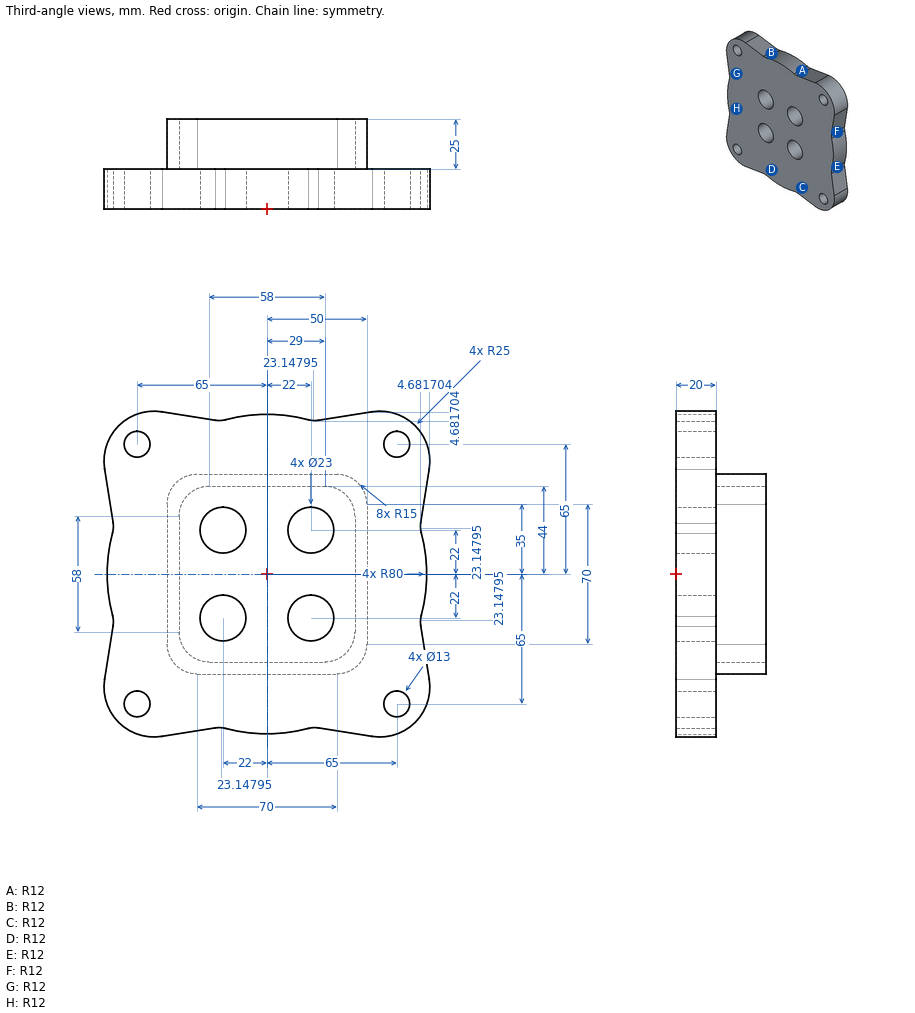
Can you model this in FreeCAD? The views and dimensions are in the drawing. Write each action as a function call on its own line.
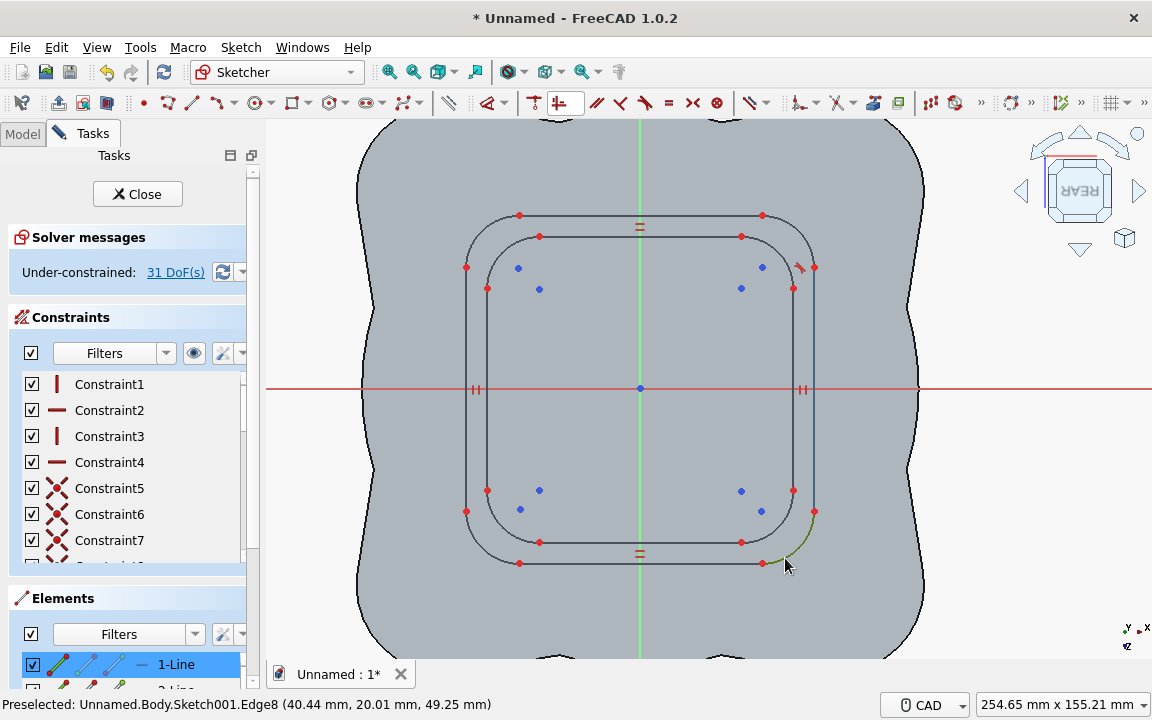
click(646, 104)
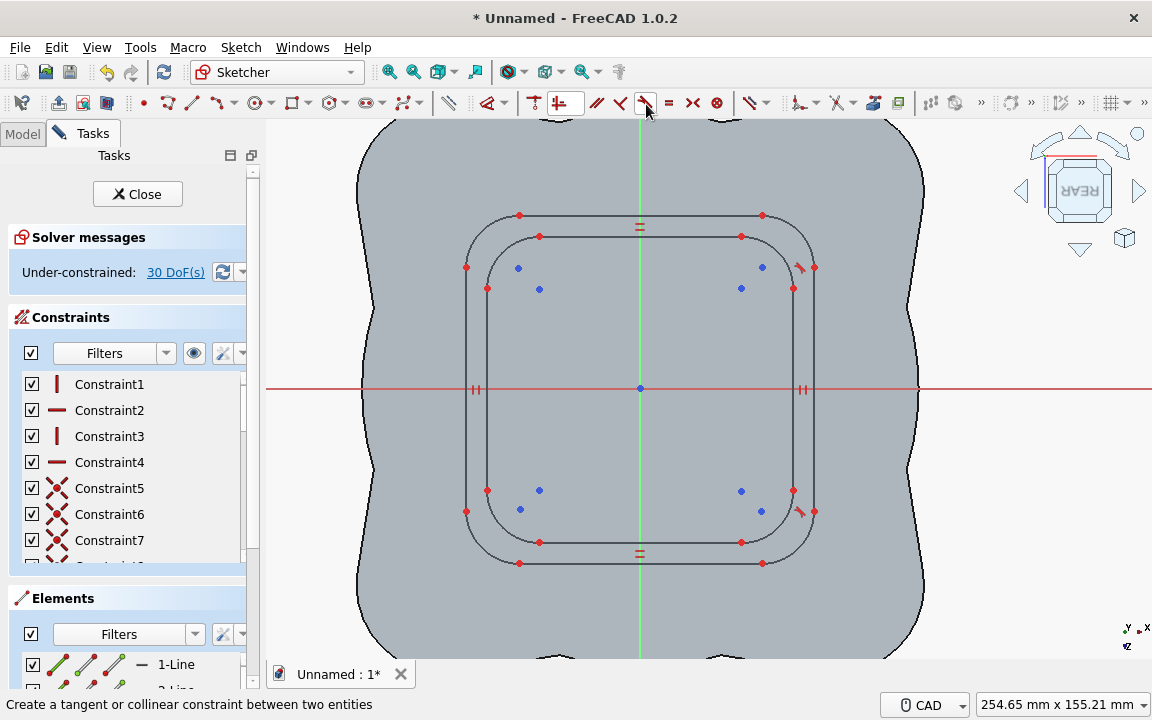
click(689, 216)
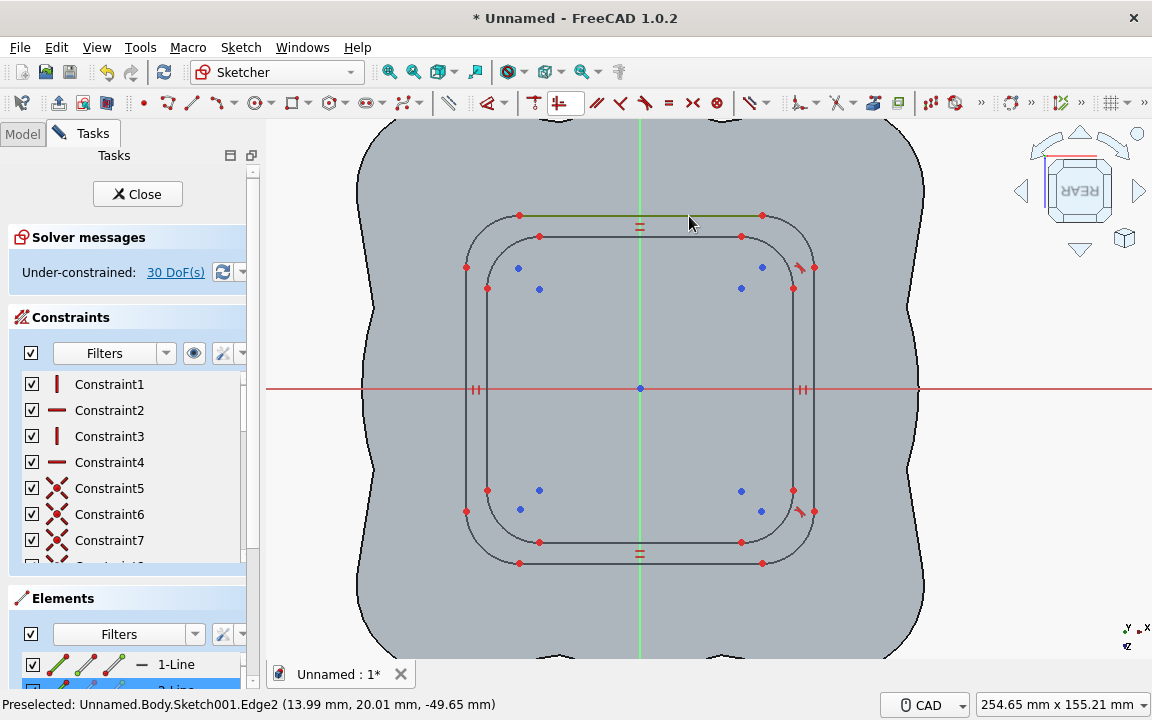
click(808, 244)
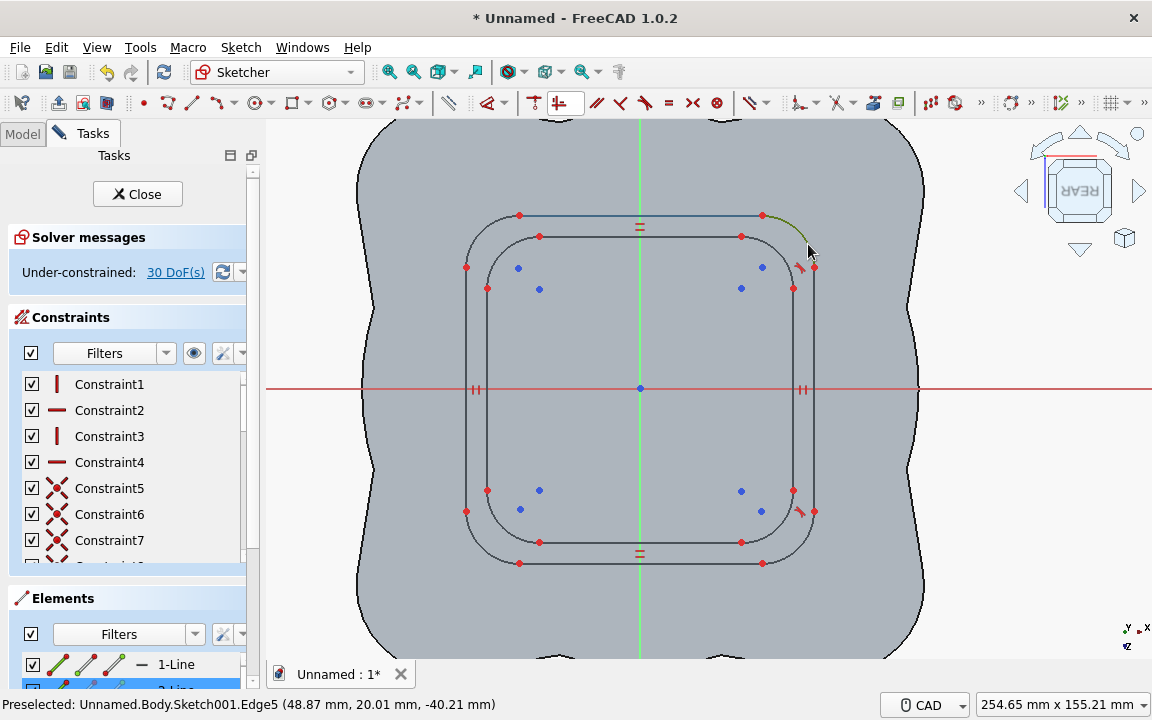
click(646, 104)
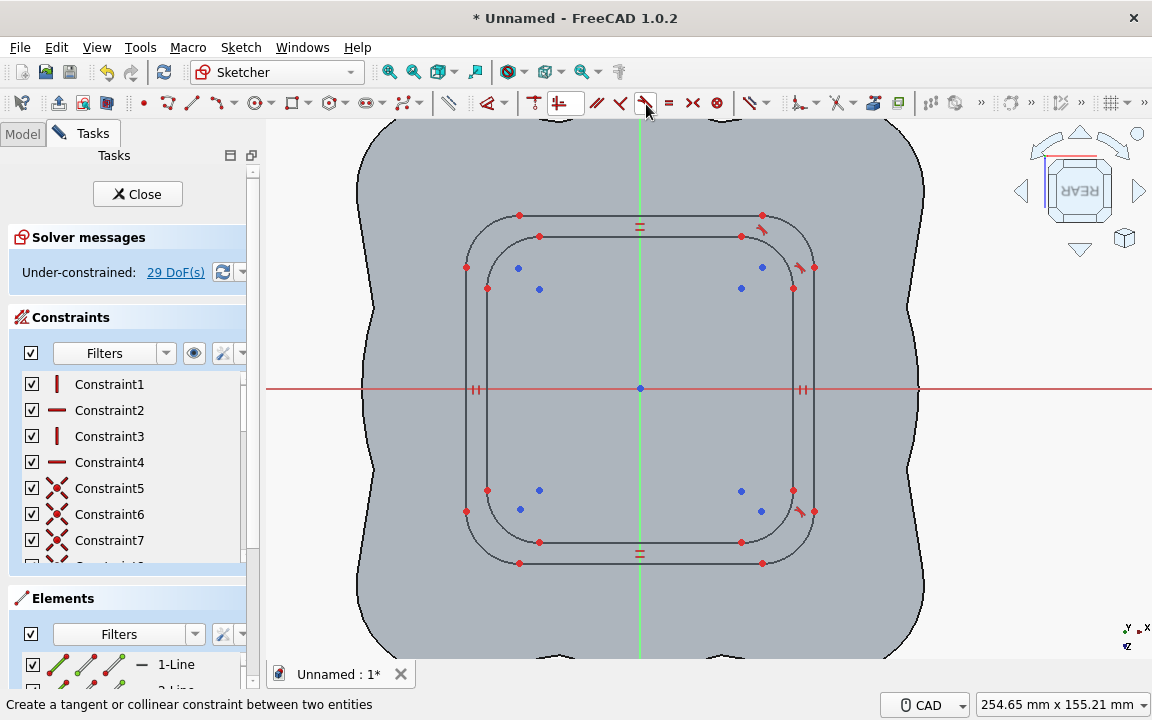
click(689, 216)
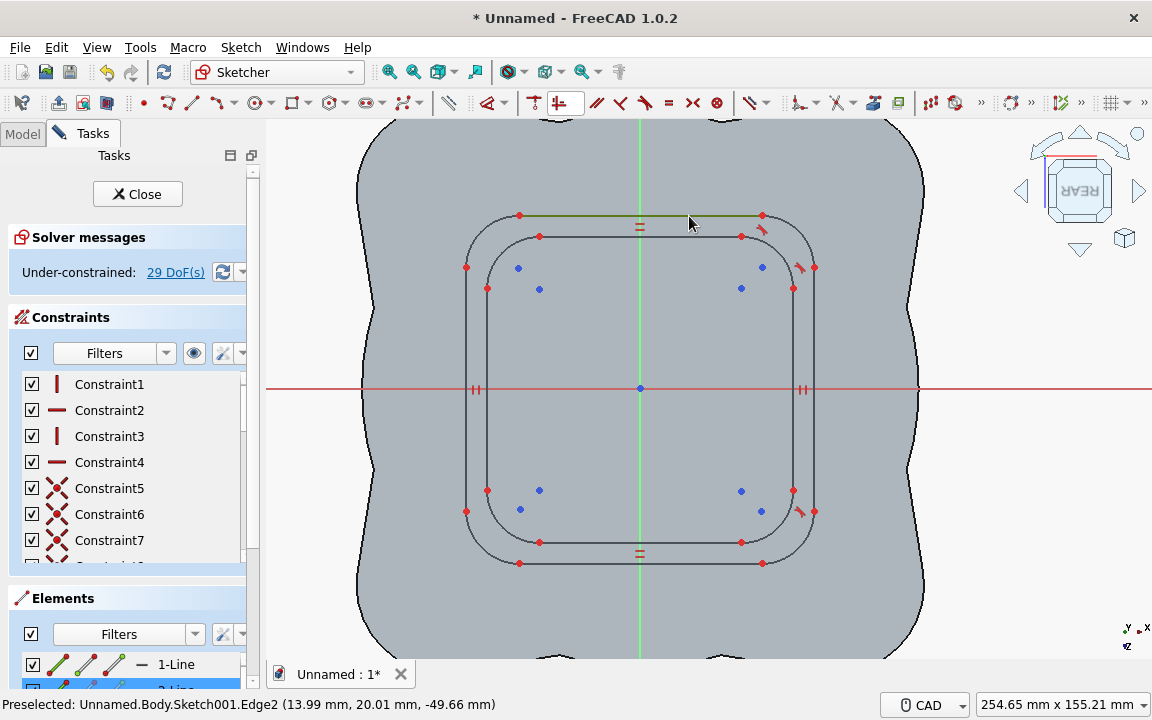
click(495, 222)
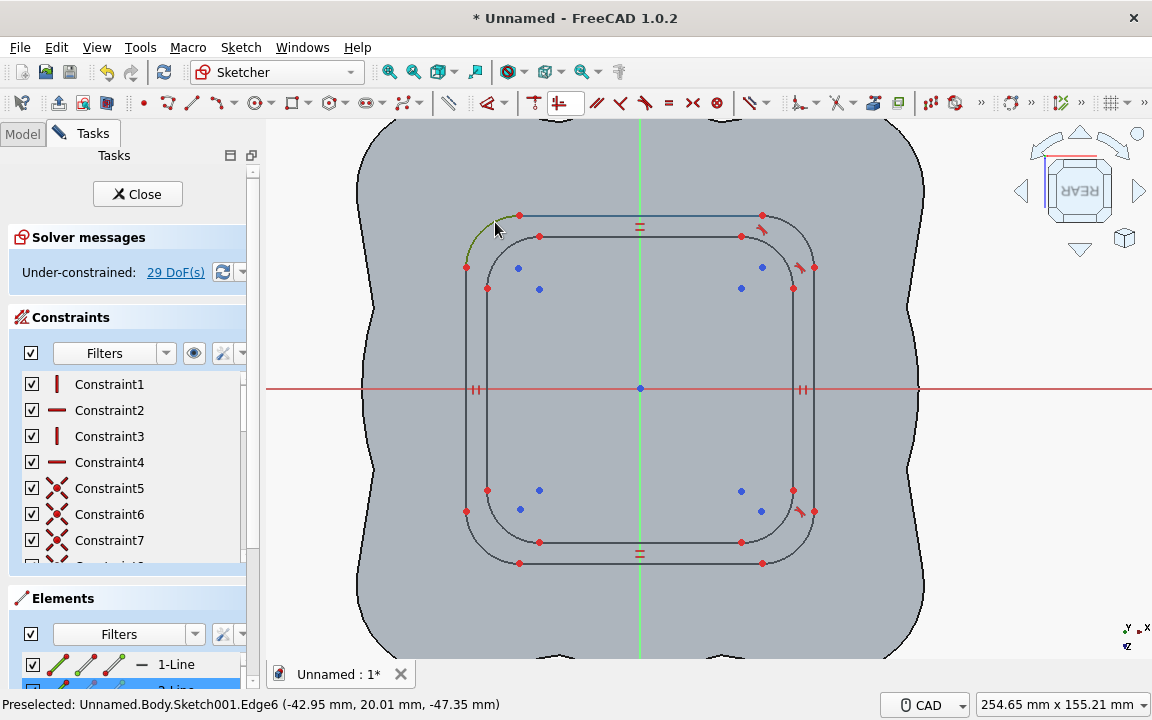
click(646, 104)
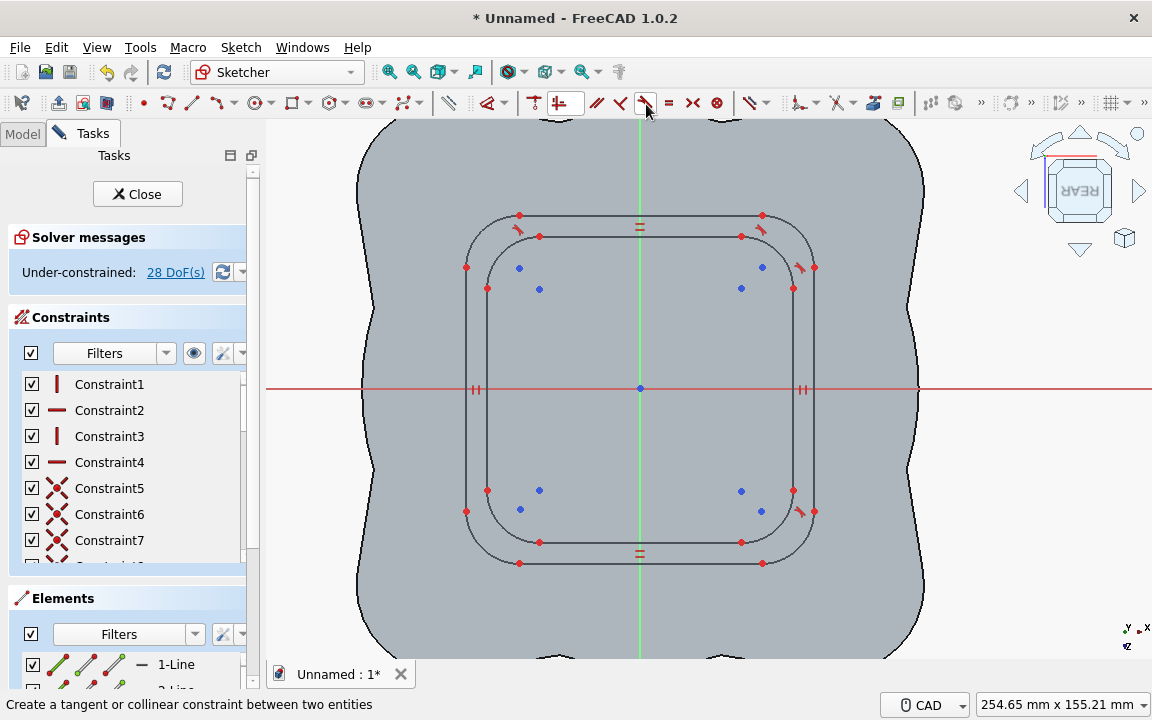
click(466, 341)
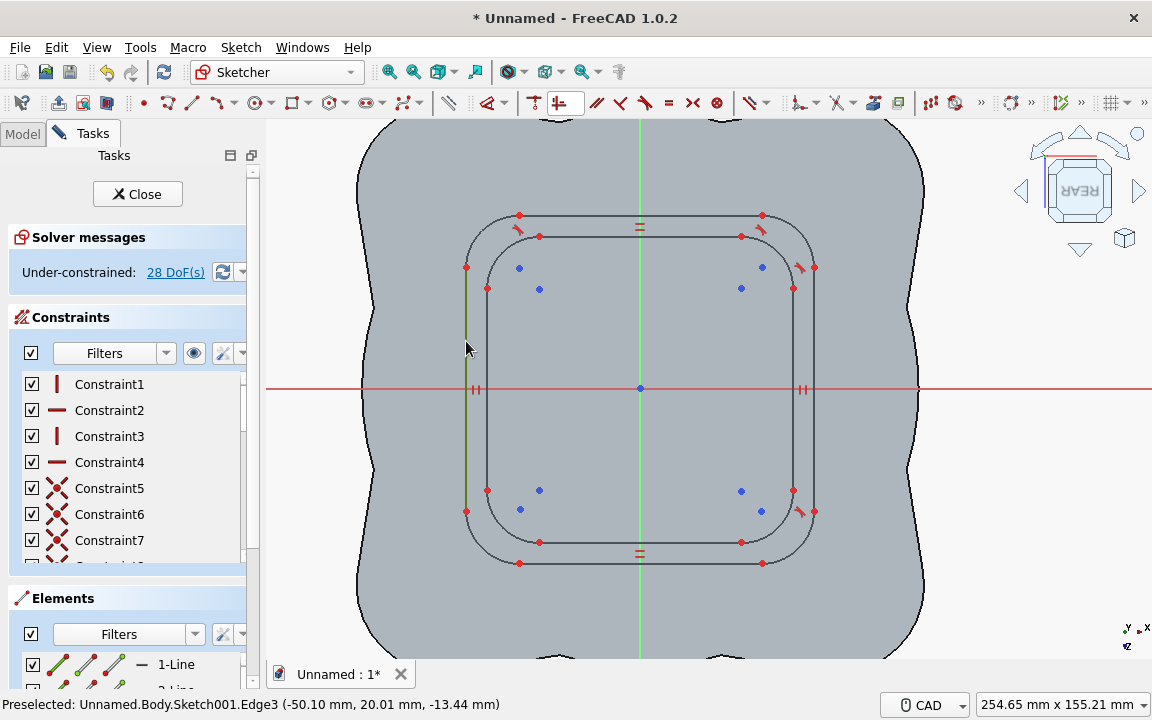
click(495, 222)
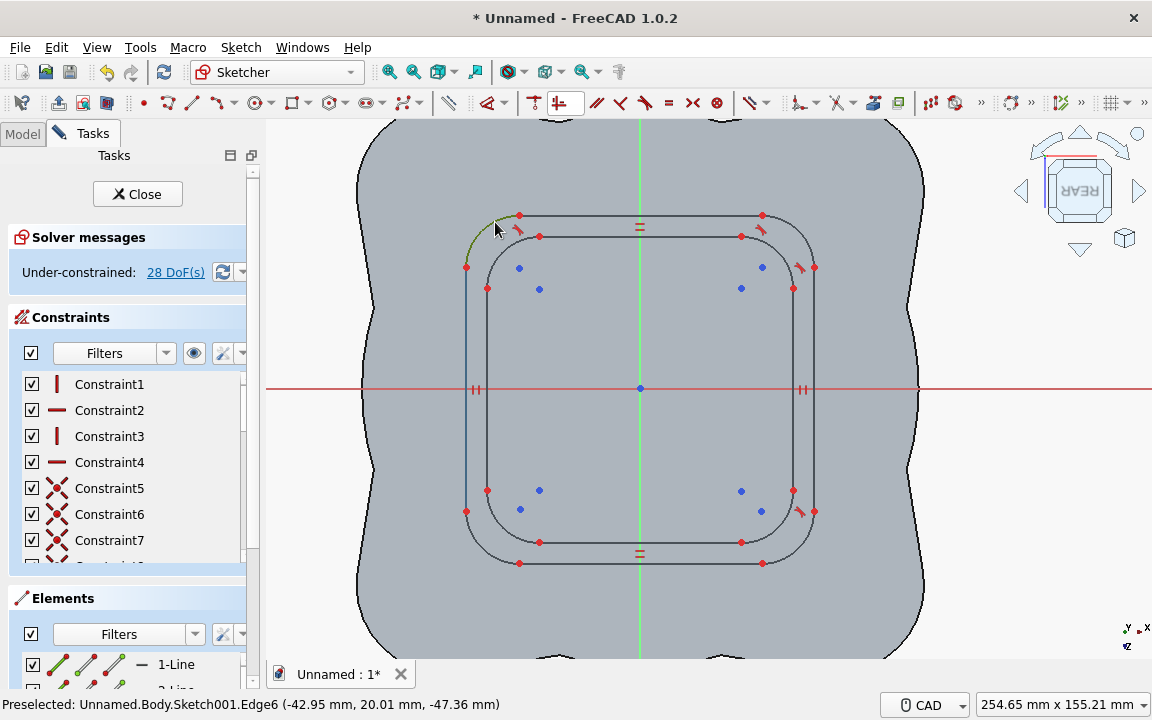
click(646, 104)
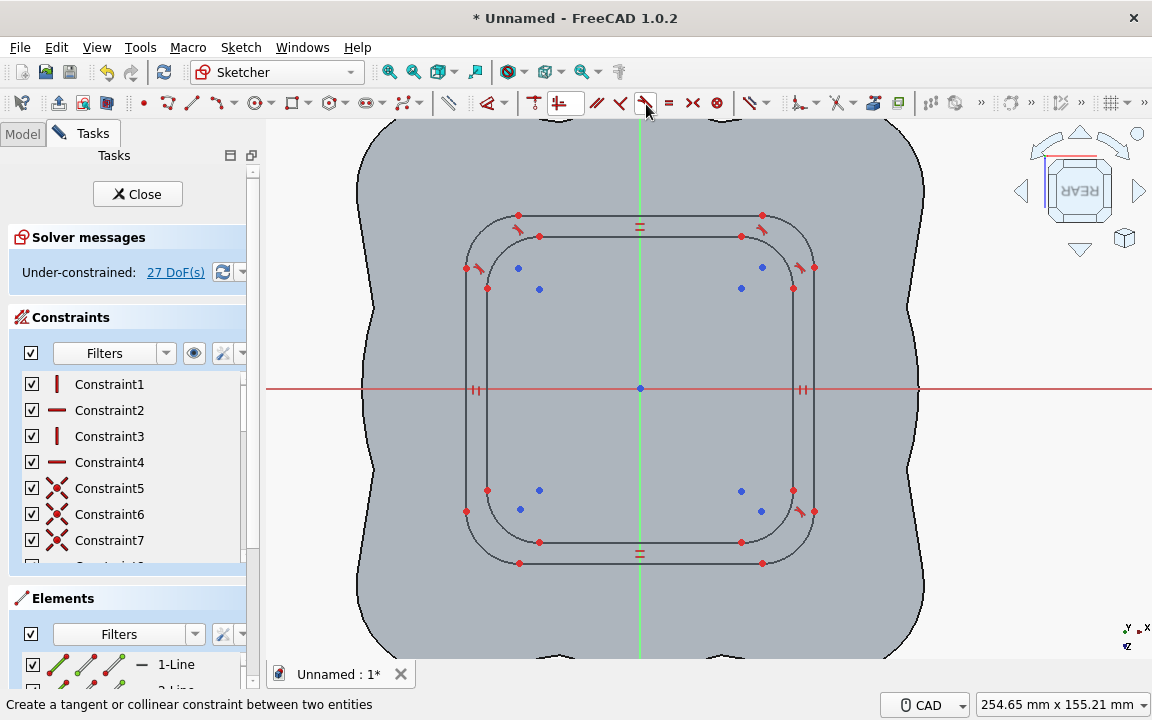
click(466, 342)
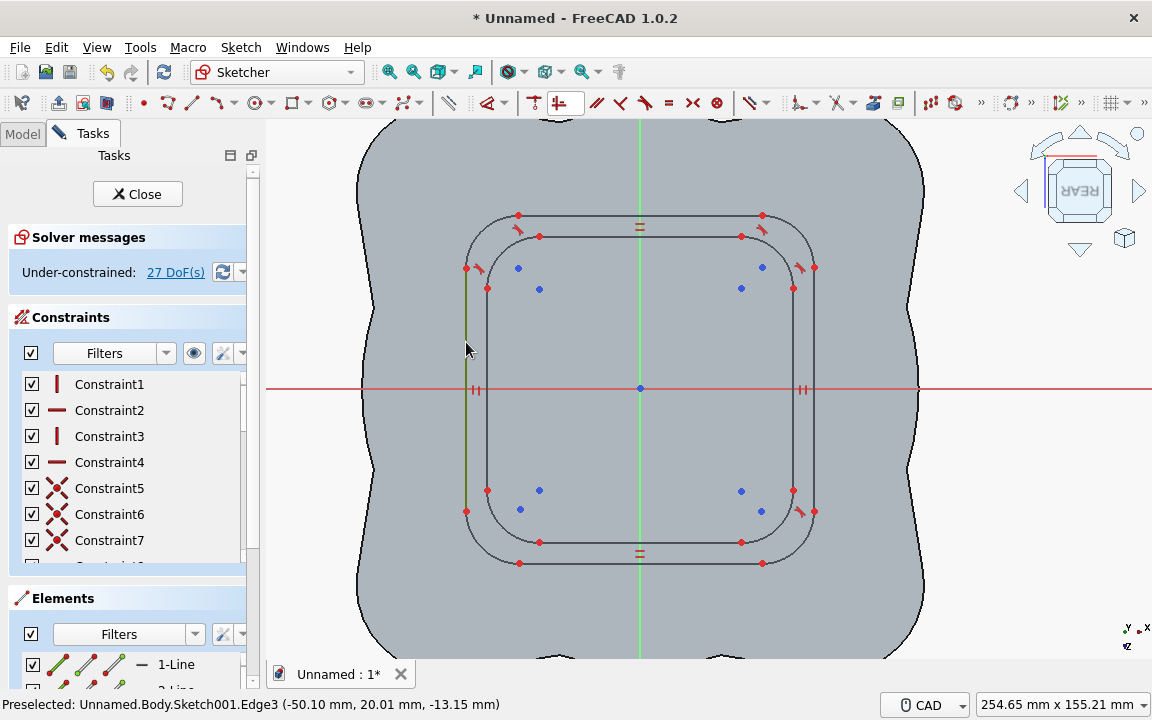
click(473, 535)